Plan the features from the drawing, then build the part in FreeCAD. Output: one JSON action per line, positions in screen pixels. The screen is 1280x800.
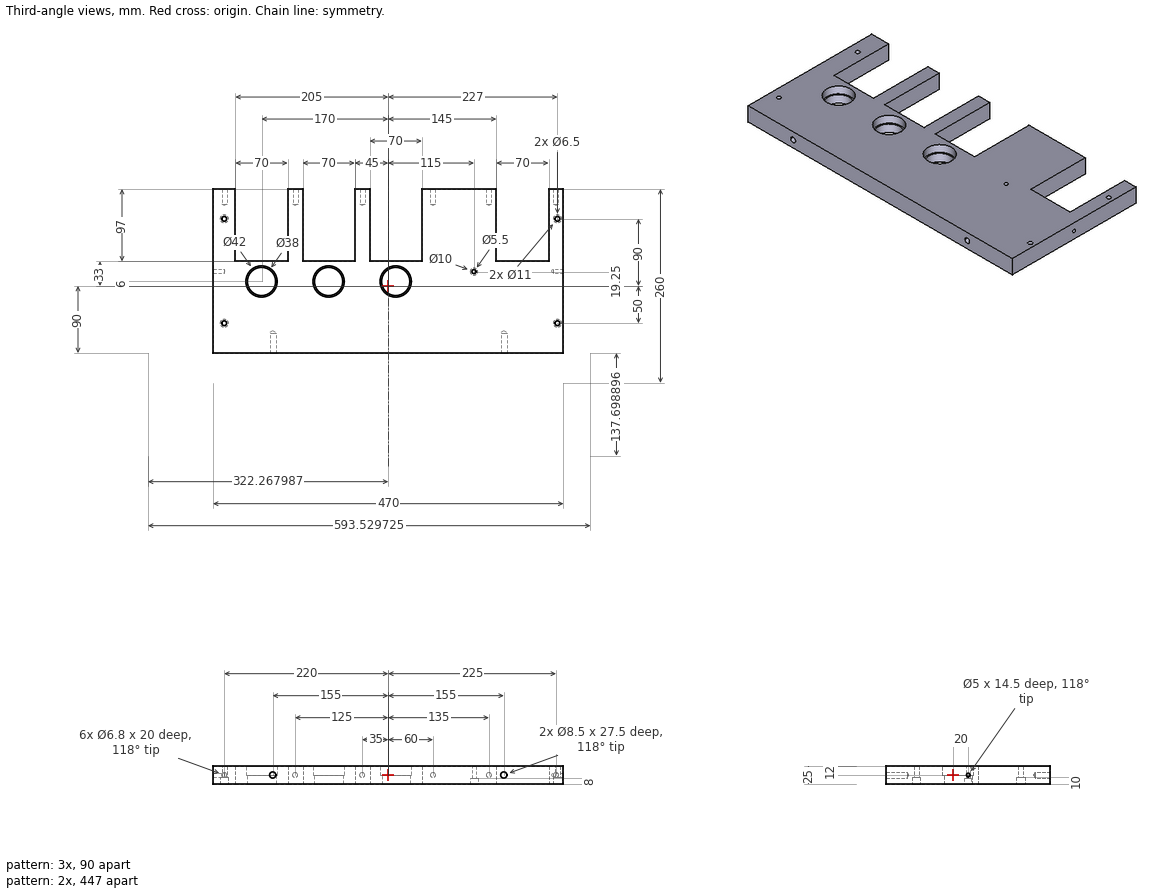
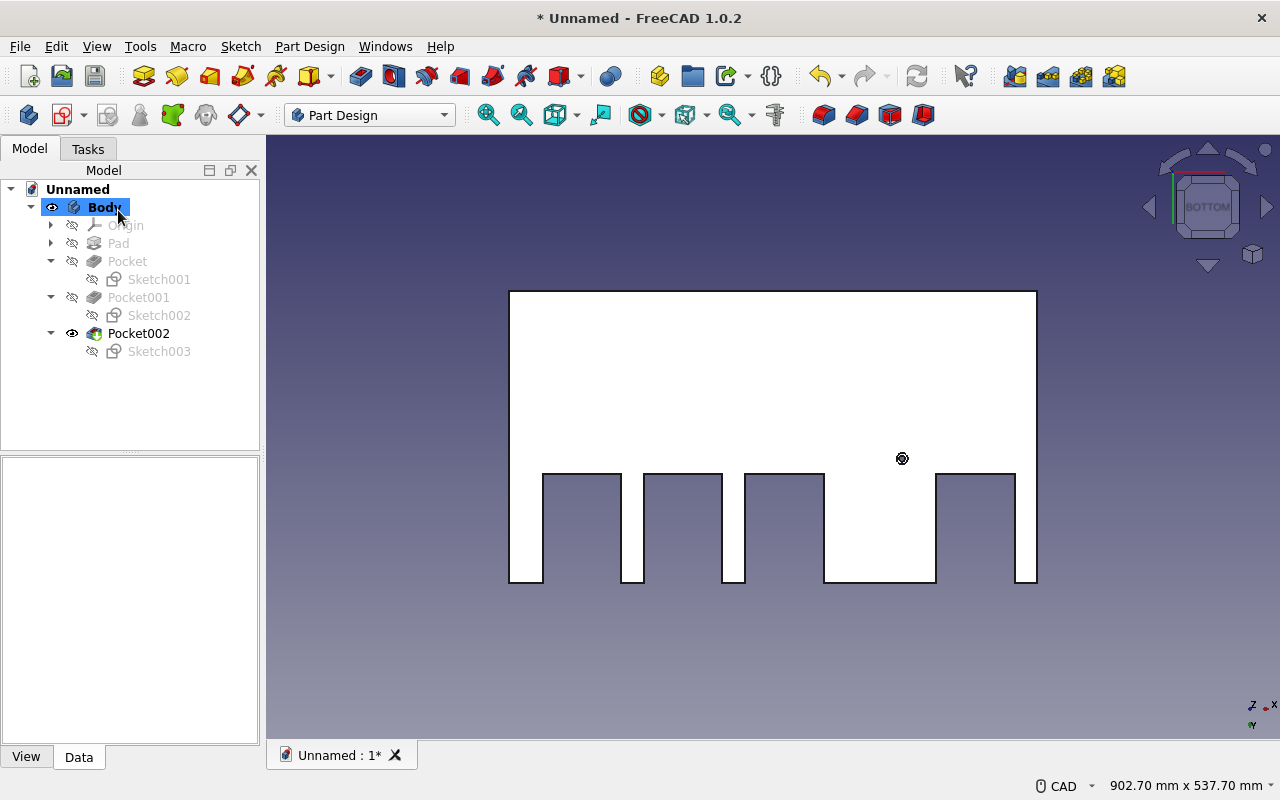
{"action": "left_click", "coordinate": [622, 394]}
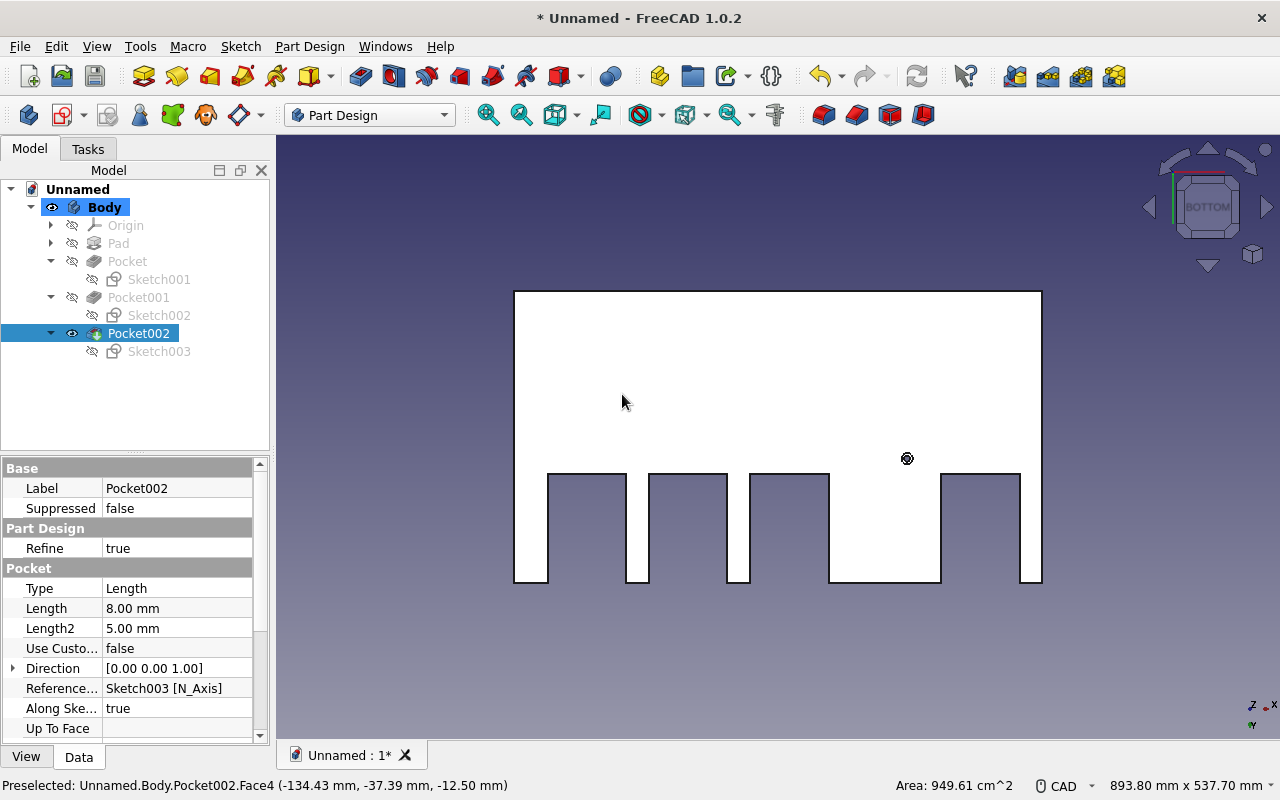
{"action": "left_click", "coordinate": [62, 116]}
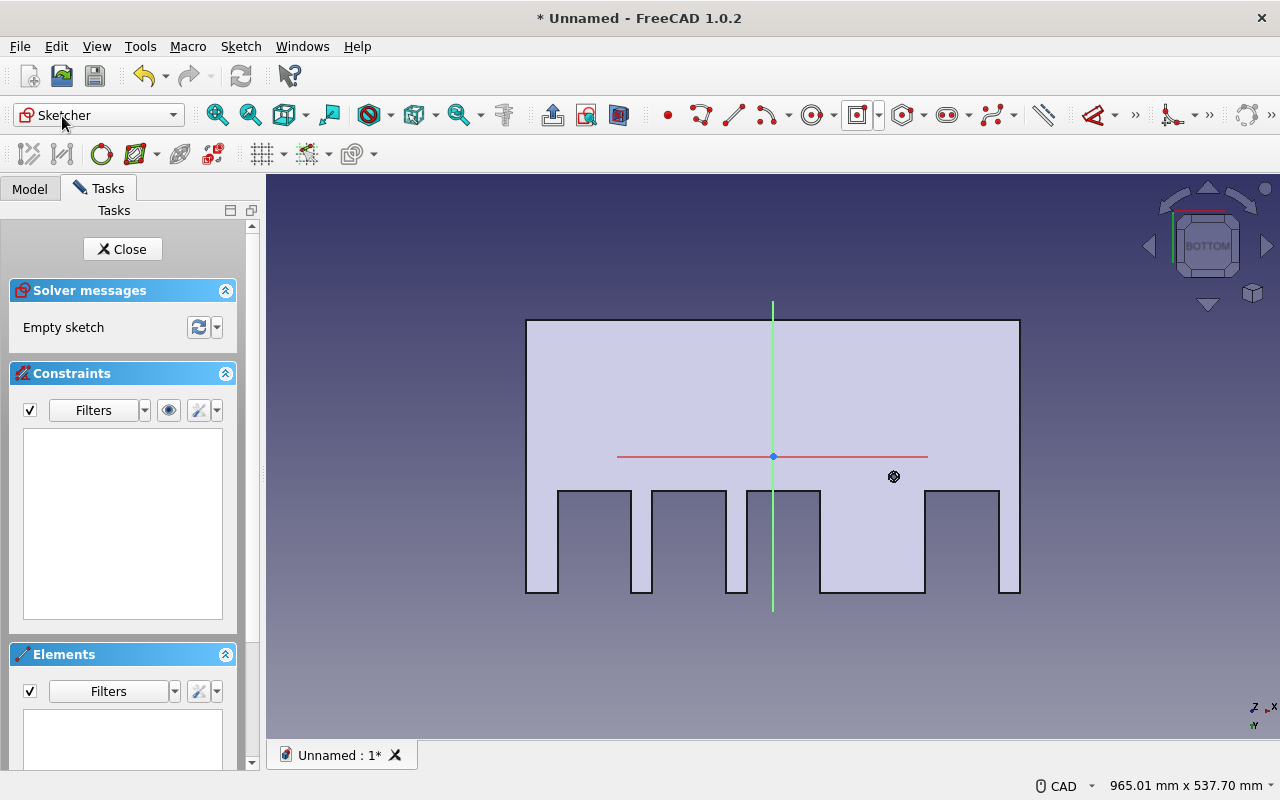
{"action": "scroll", "coordinate": [516, 711], "scroll_direction": "down", "scroll_amount": 1}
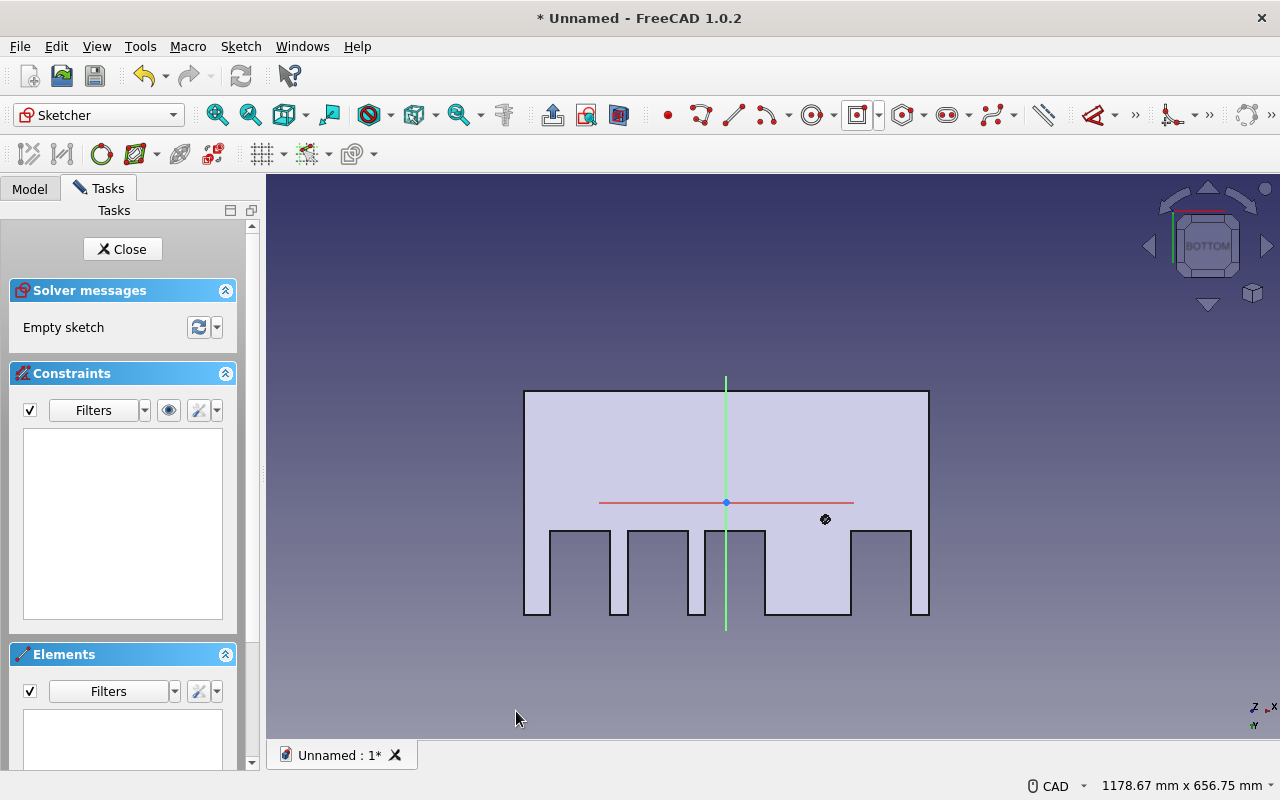
{"action": "left_click", "coordinate": [878, 116]}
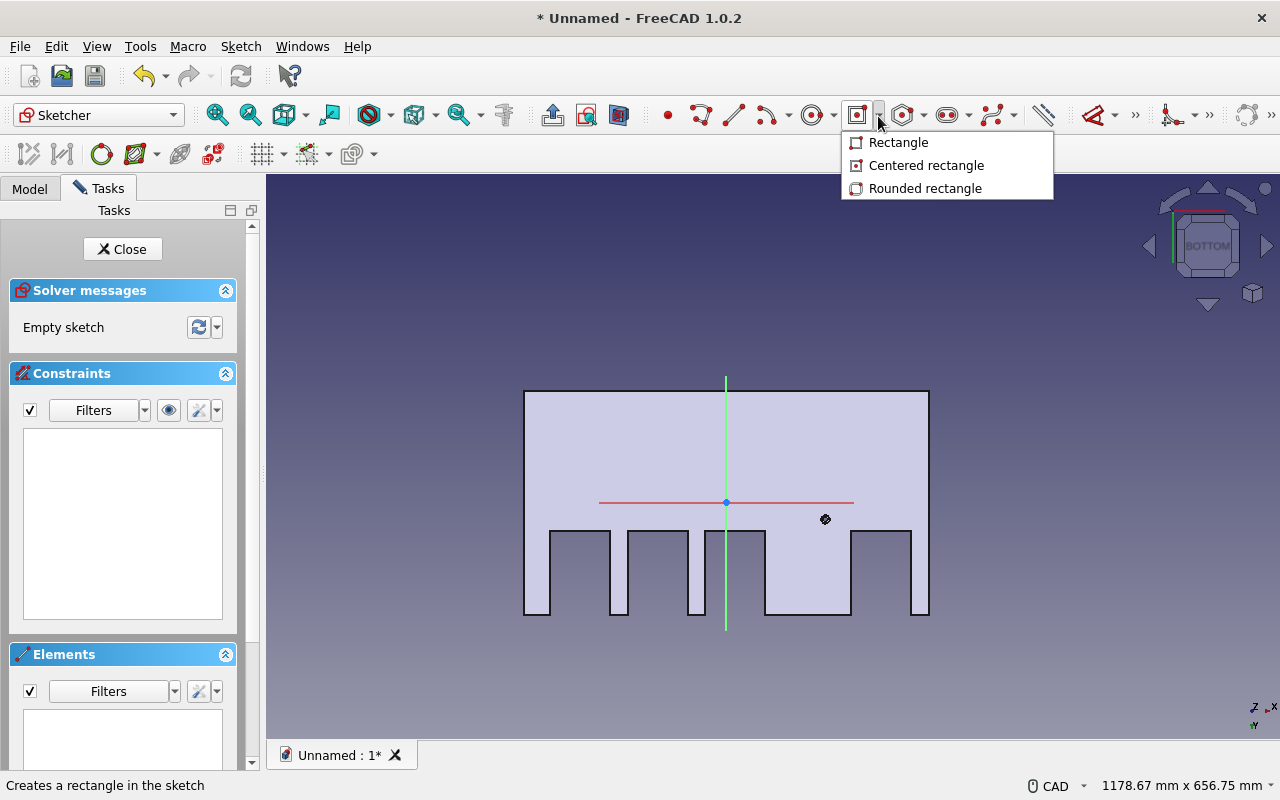
{"action": "left_click", "coordinate": [948, 142]}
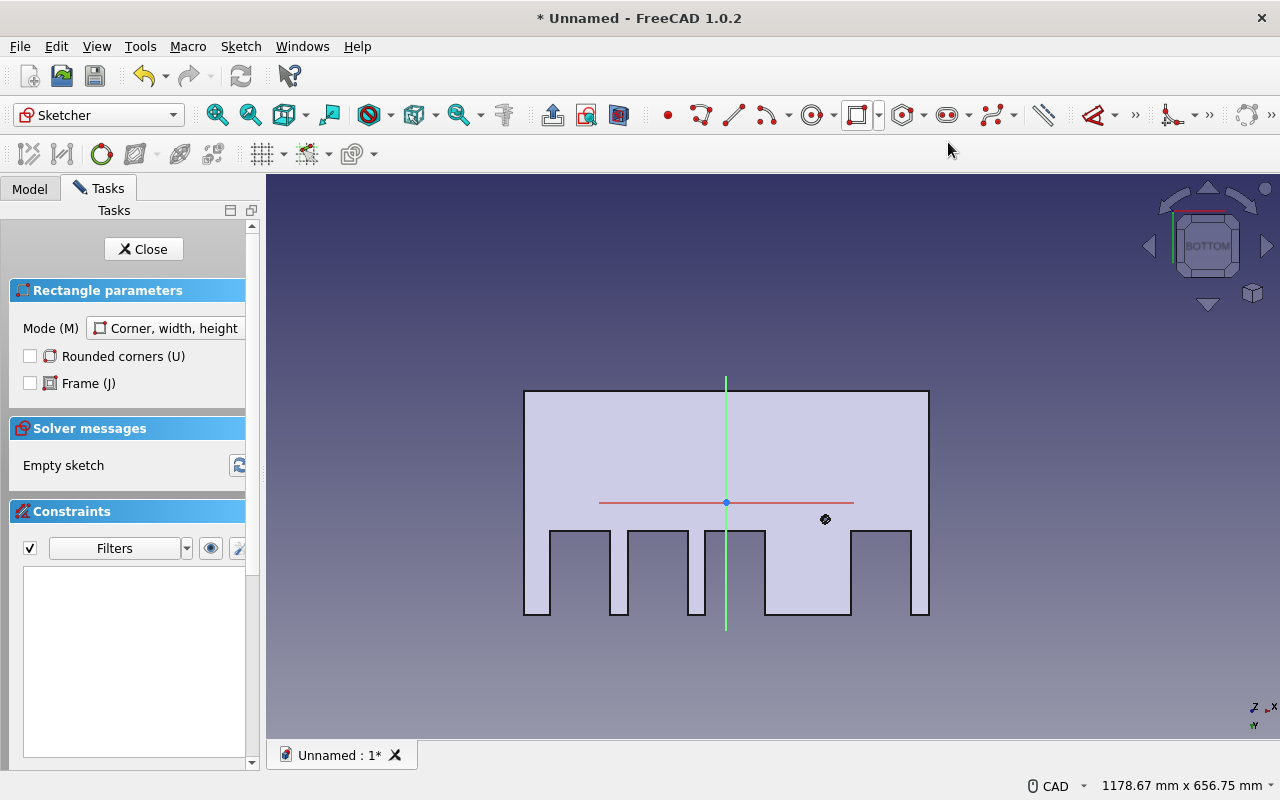
{"action": "left_click", "coordinate": [449, 307]}
{"action": "mouse_move", "coordinate": [960, 425]}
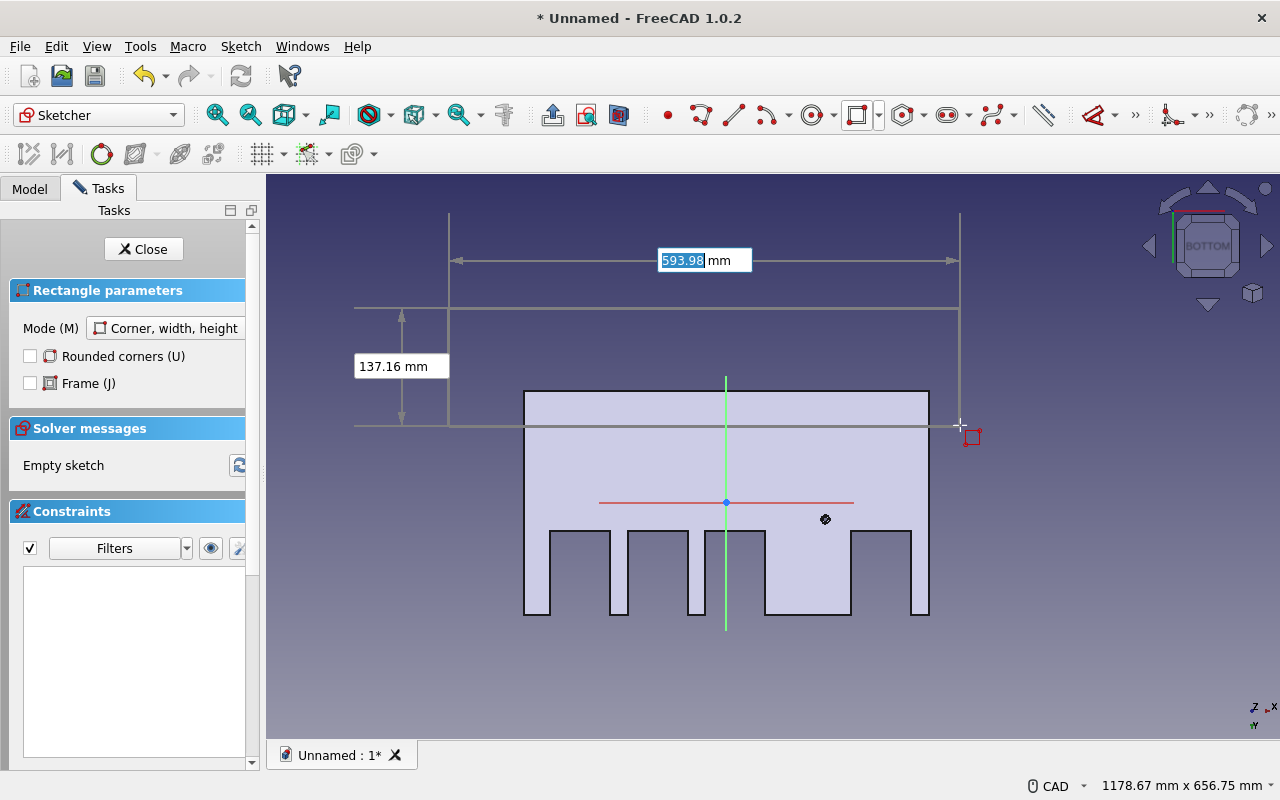
{"action": "type", "text": "593.529725"}
{"action": "key", "text": "Tab"}
{"action": "type", "text": "137.698896"}
{"action": "key", "text": "Return"}
{"action": "key", "text": "Escape"}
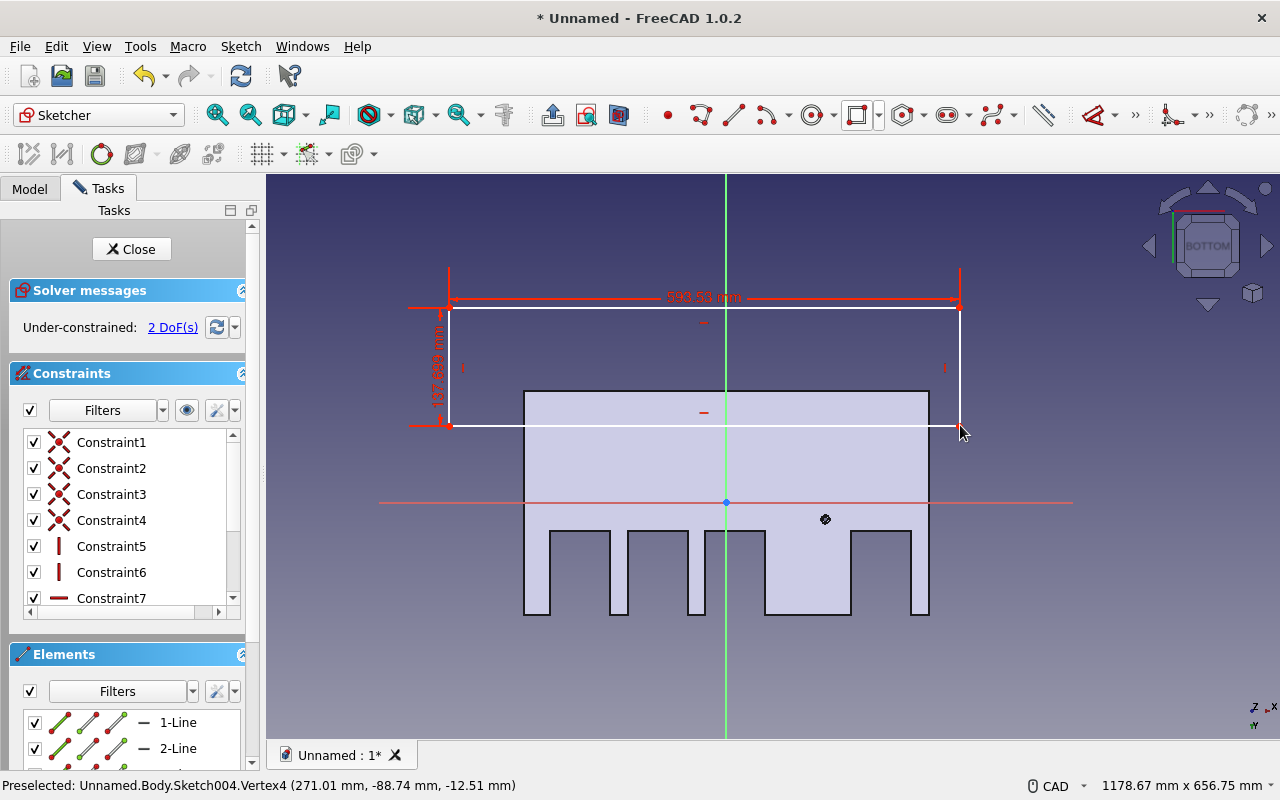
{"action": "left_click", "coordinate": [1092, 116]}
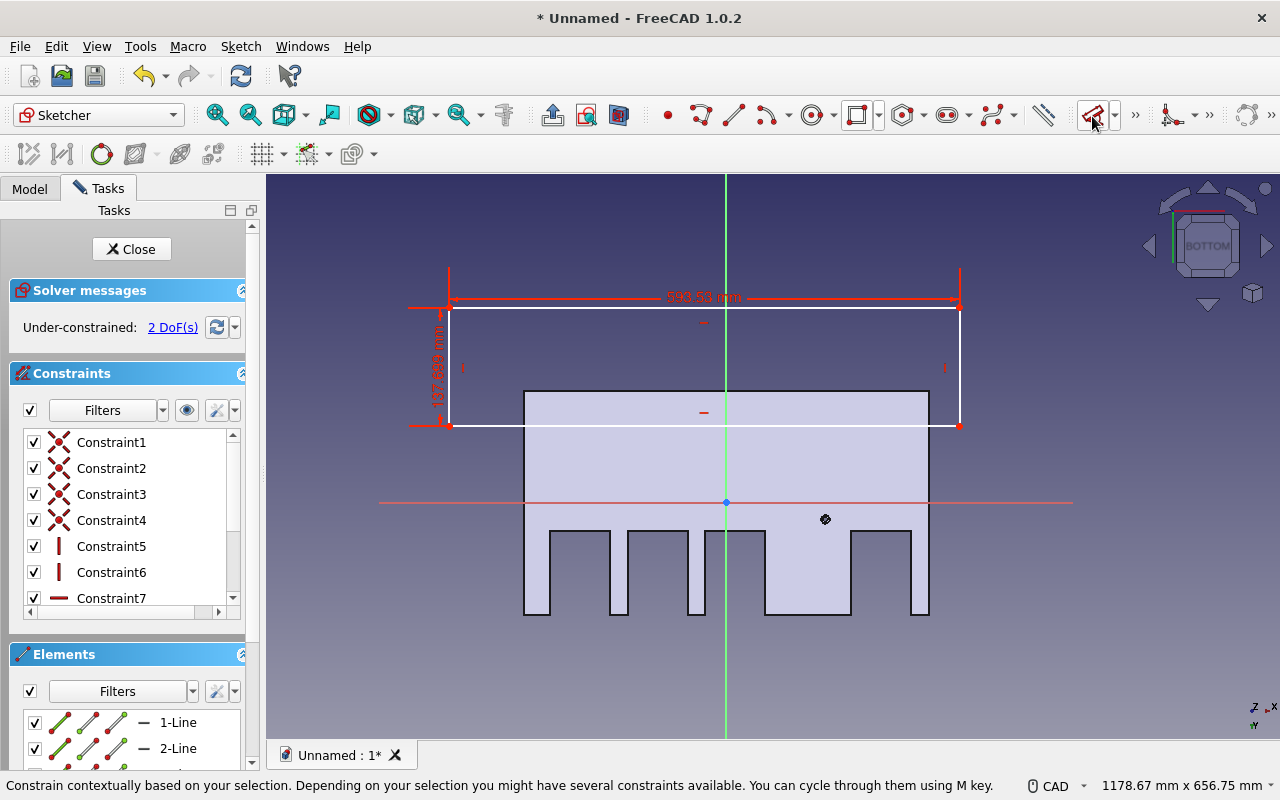
{"action": "left_click", "coordinate": [449, 426]}
{"action": "left_click", "coordinate": [415, 465]}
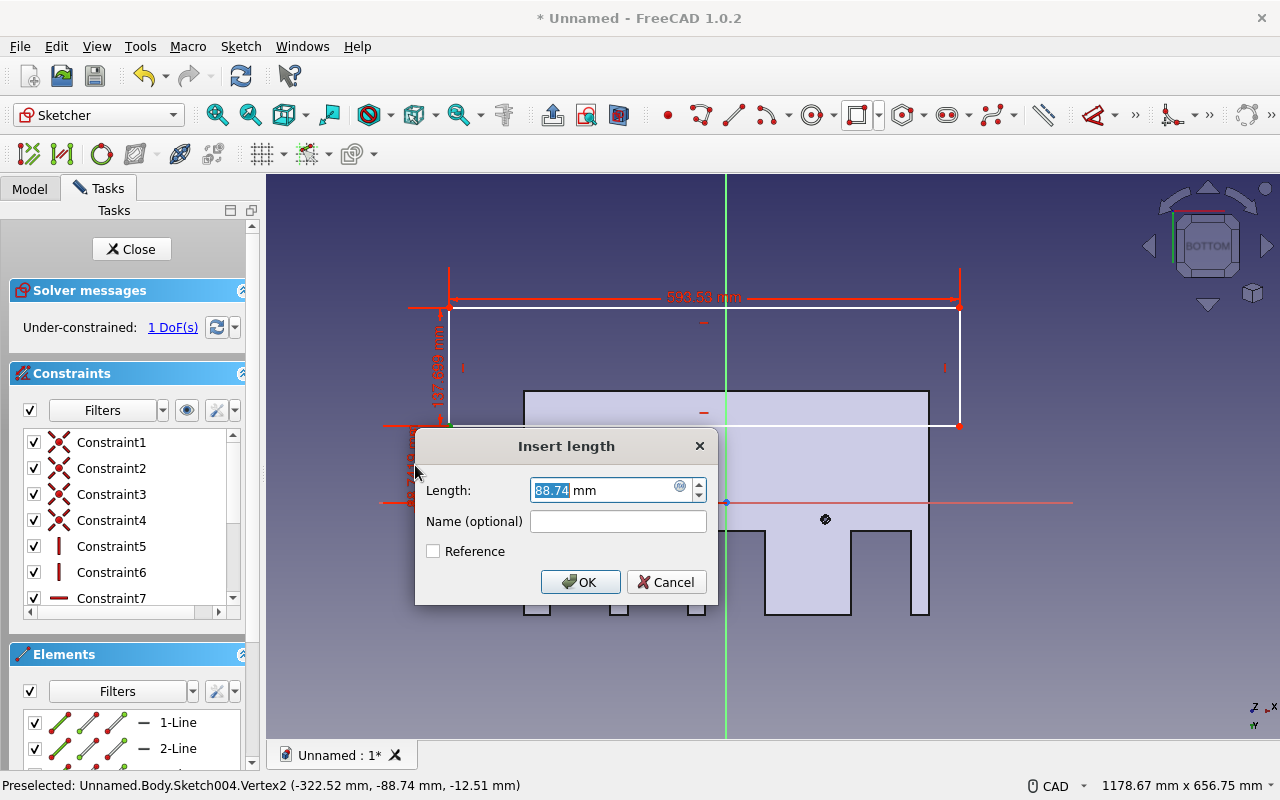
{"action": "type", "text": "90"}
{"action": "key", "text": "Return"}